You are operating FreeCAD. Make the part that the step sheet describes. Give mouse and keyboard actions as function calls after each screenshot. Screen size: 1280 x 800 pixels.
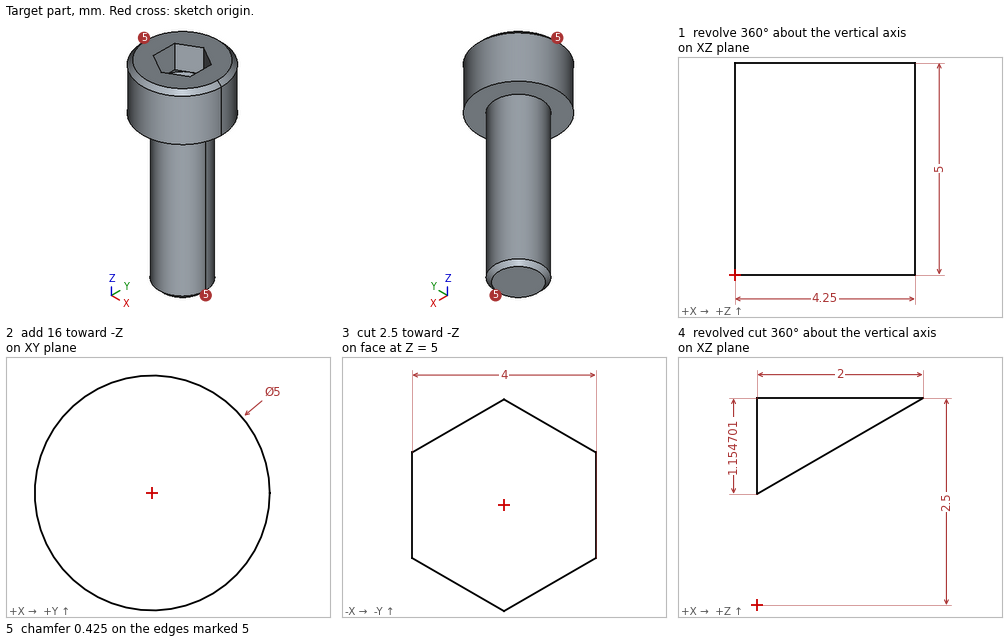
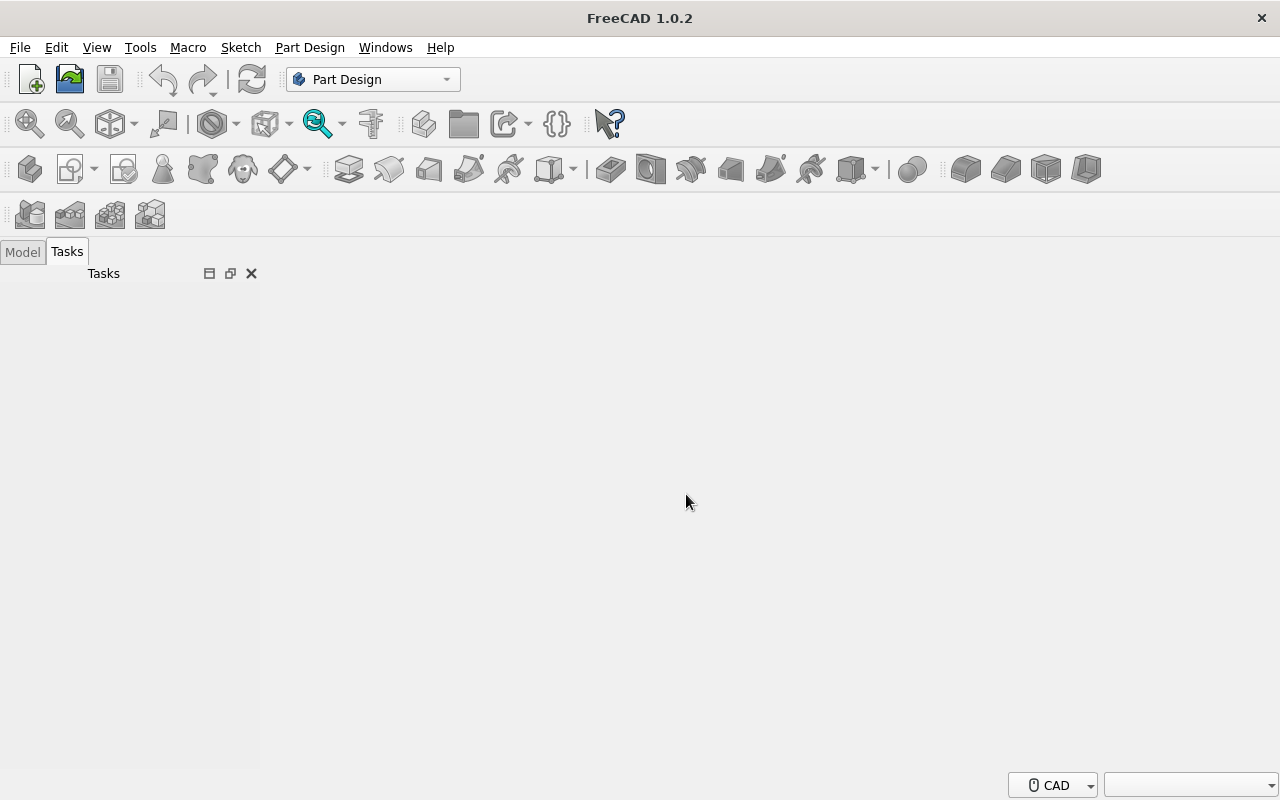
click(30, 80)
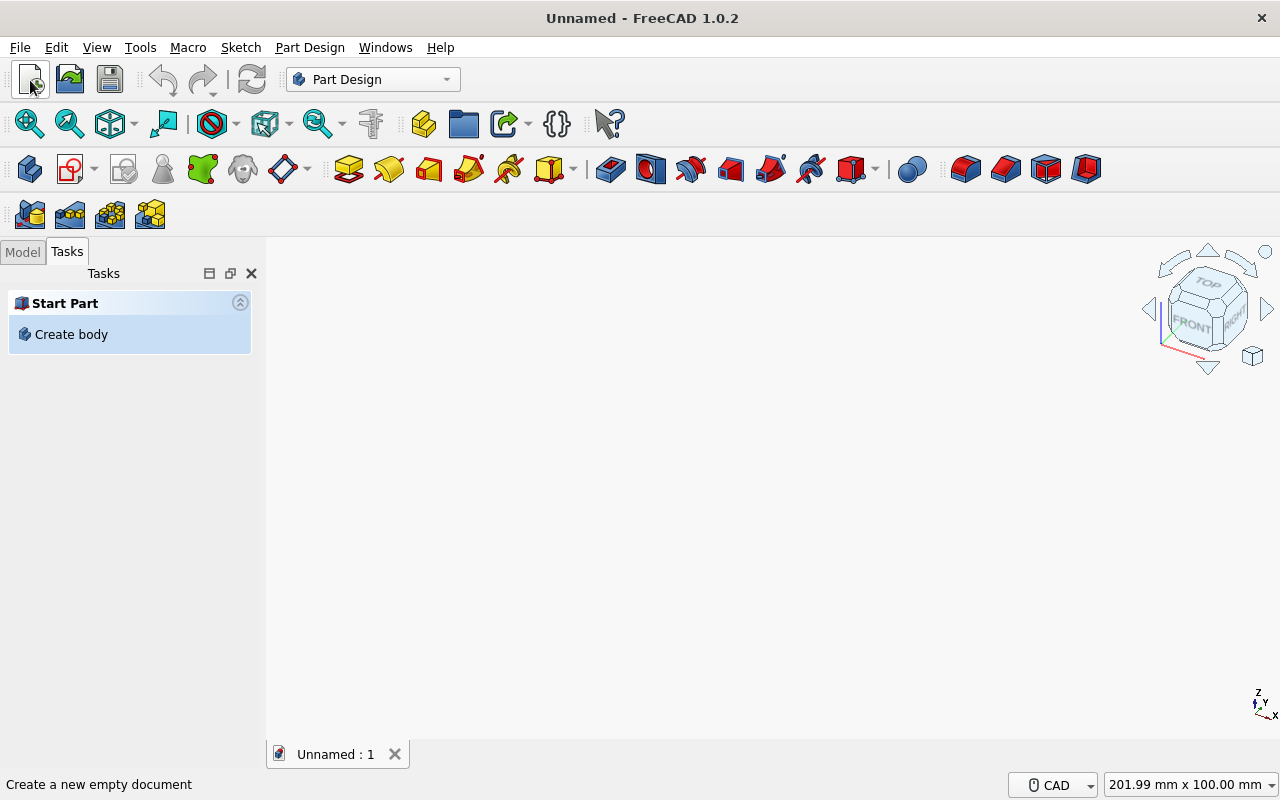
click(70, 170)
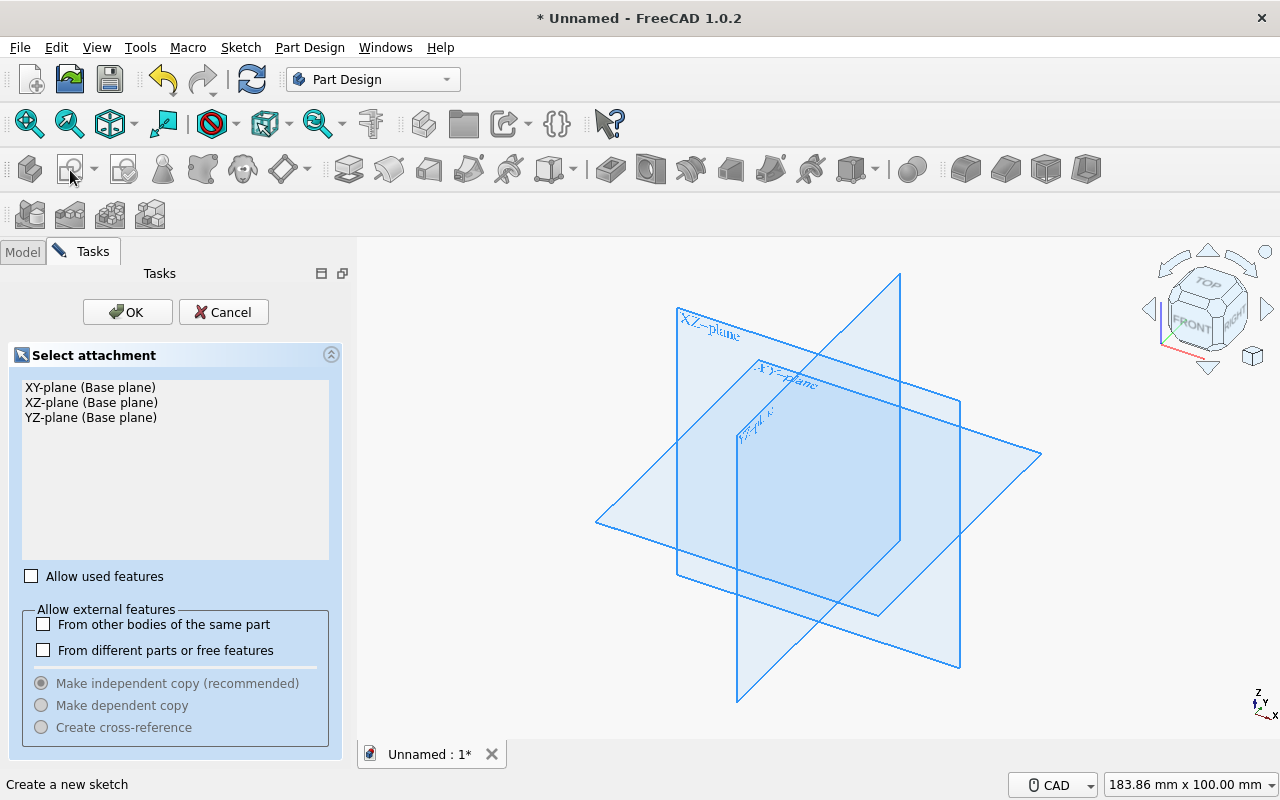
click(82, 402)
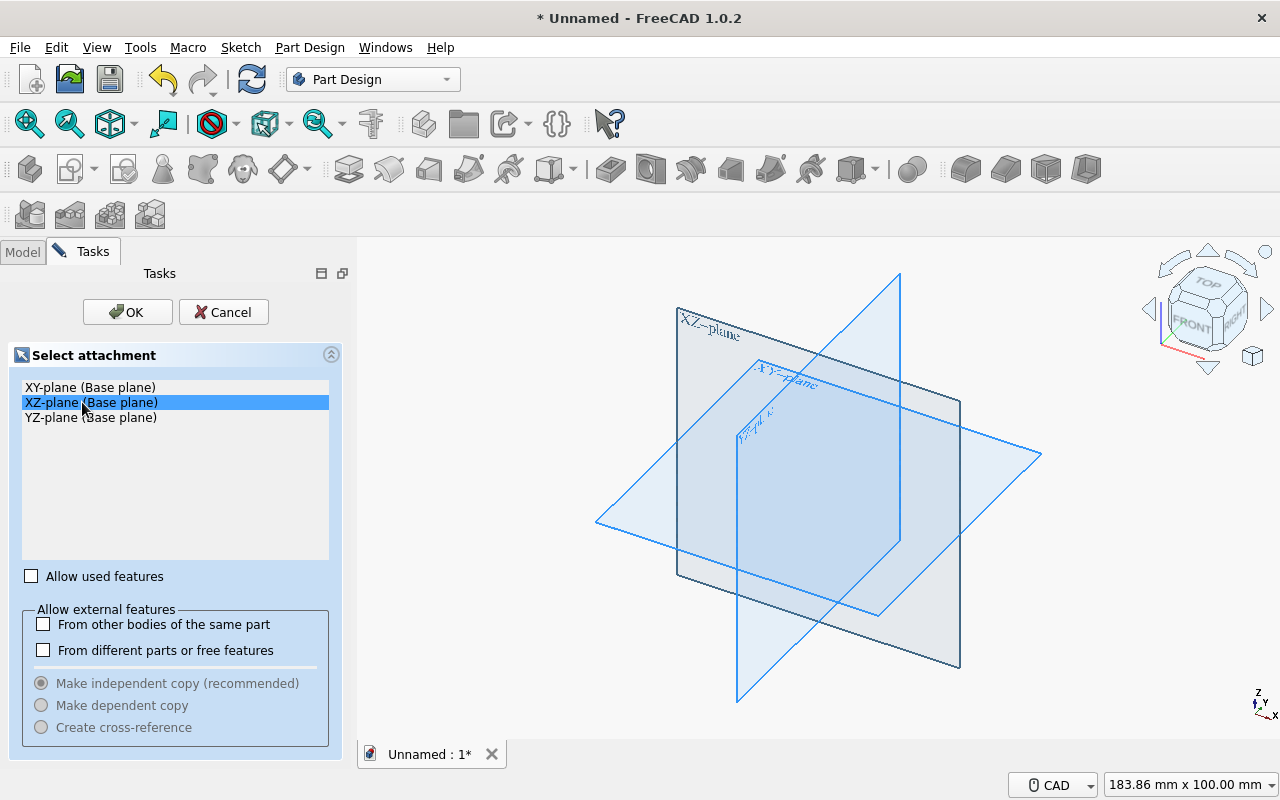
click(128, 312)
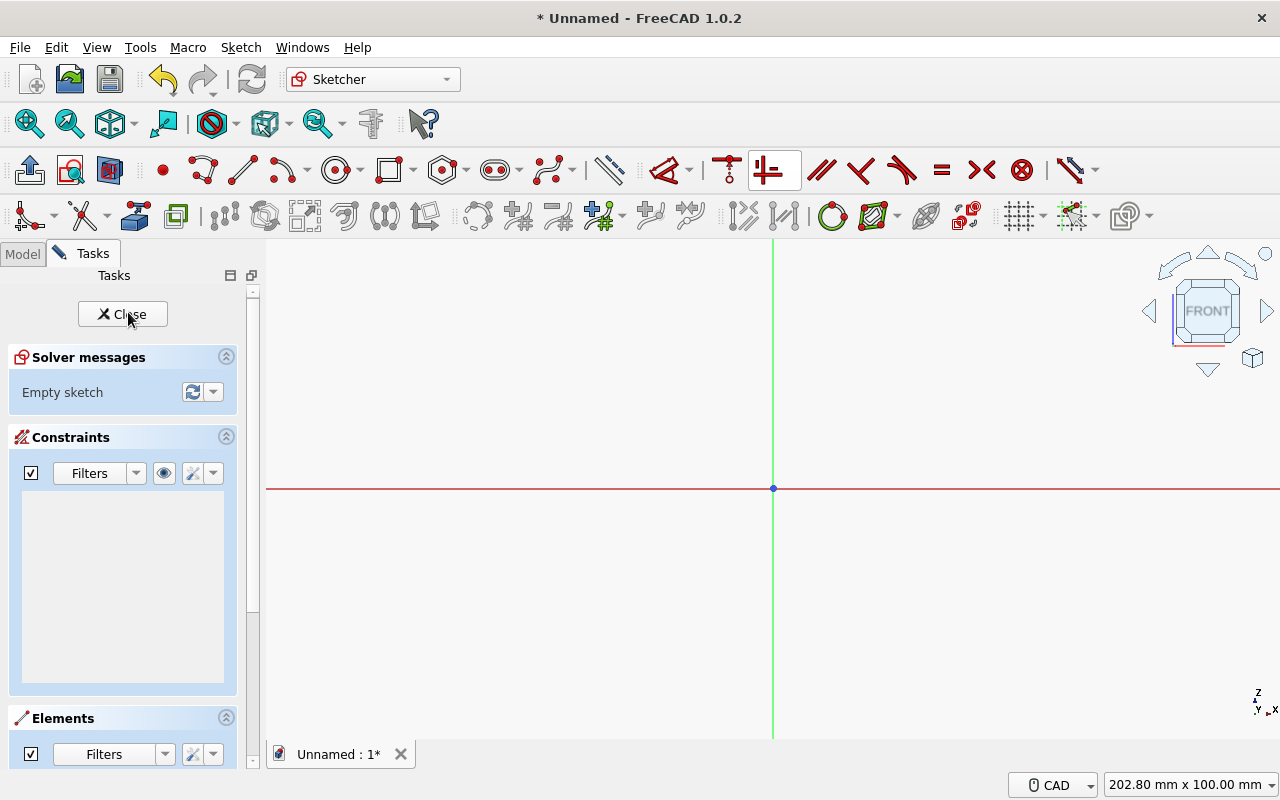
scroll(790, 475, up, 13)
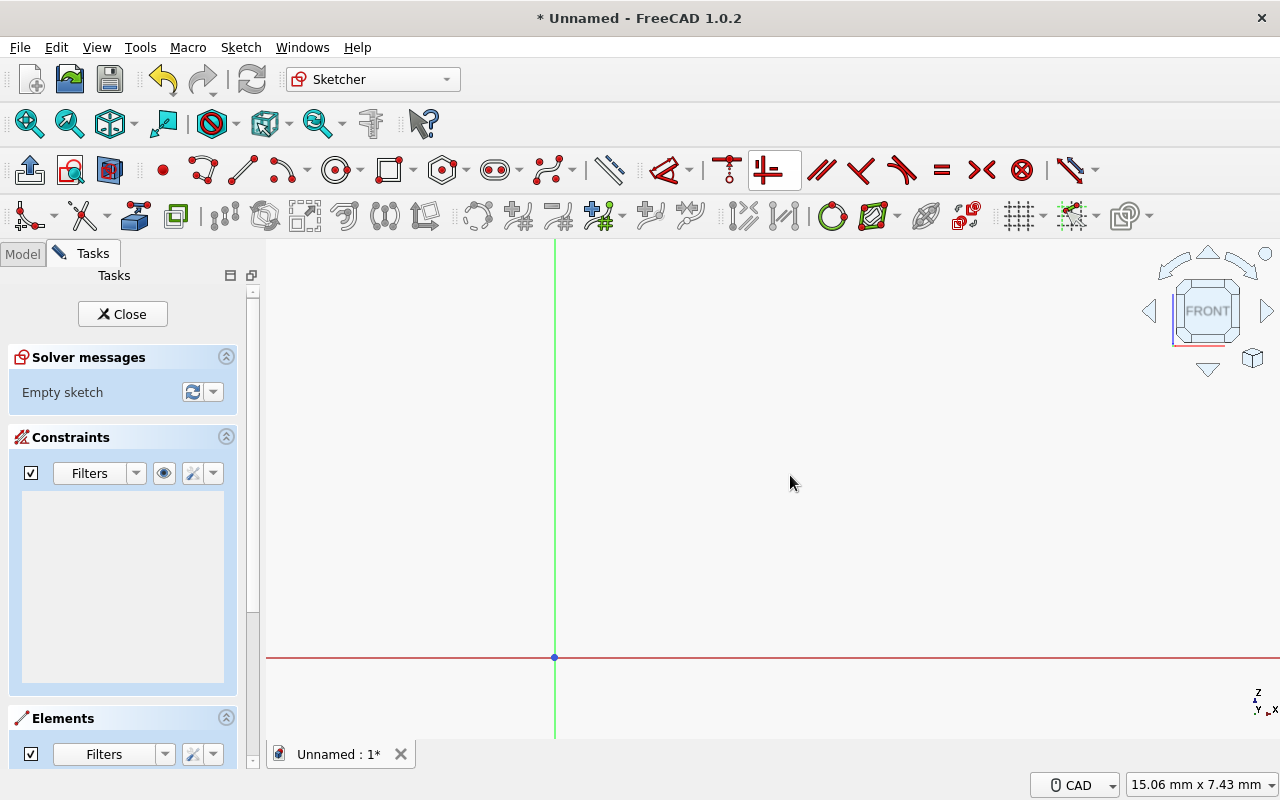
click(390, 170)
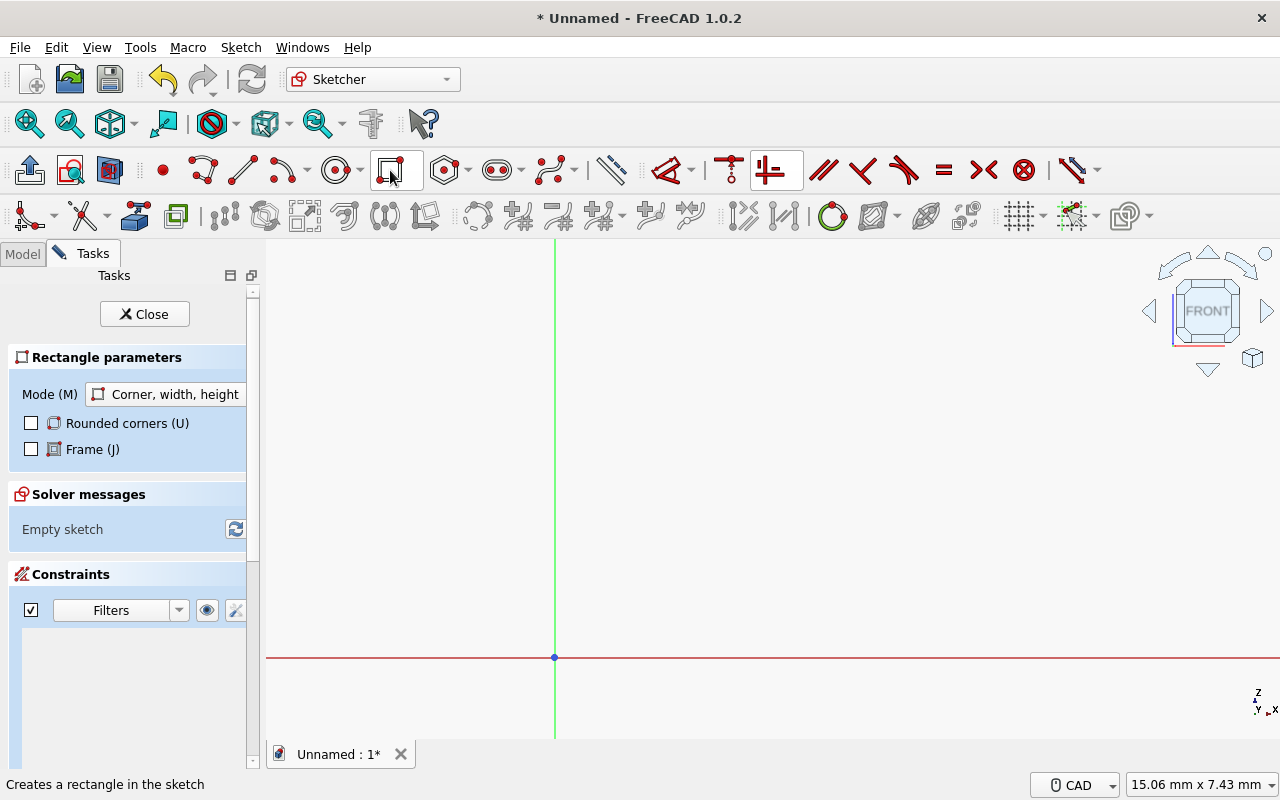
click(555, 658)
move(841, 321)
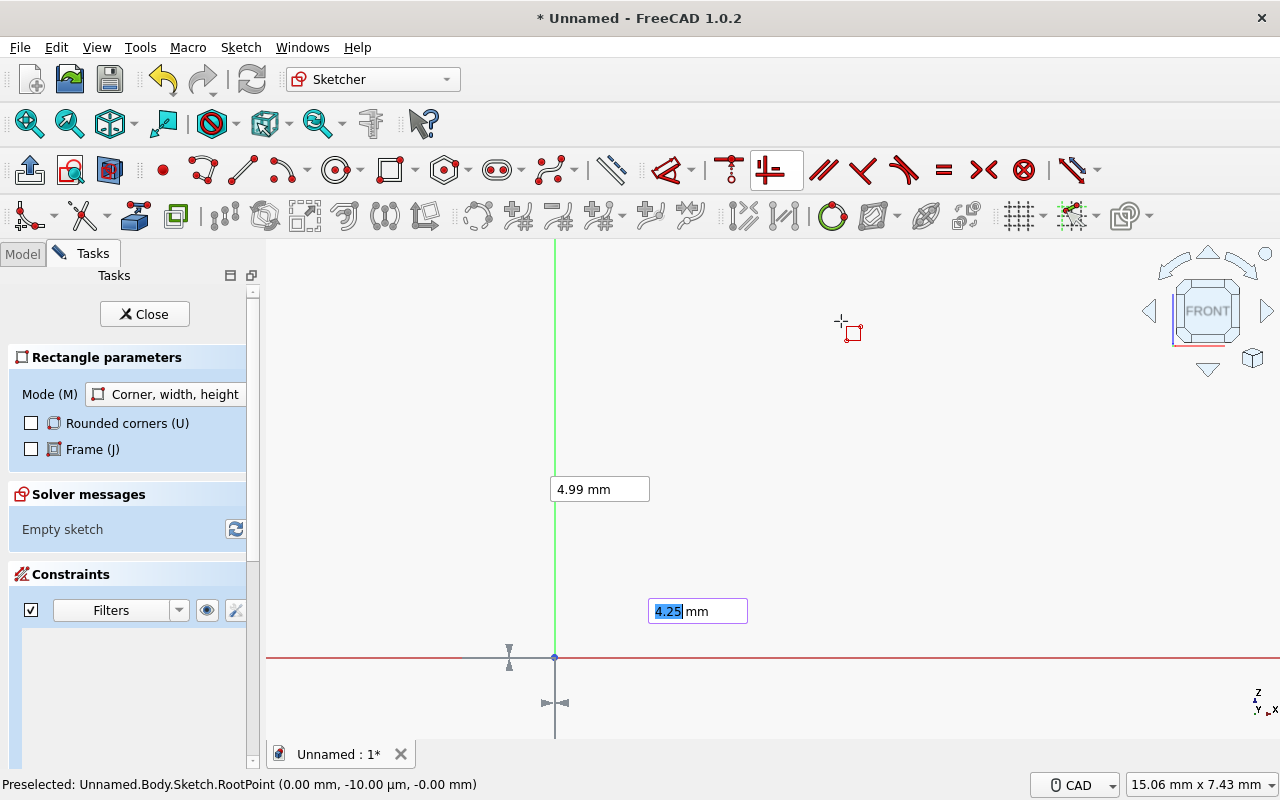
text(4.25)
key(Tab)
text(5)
key(Return)
key(Escape)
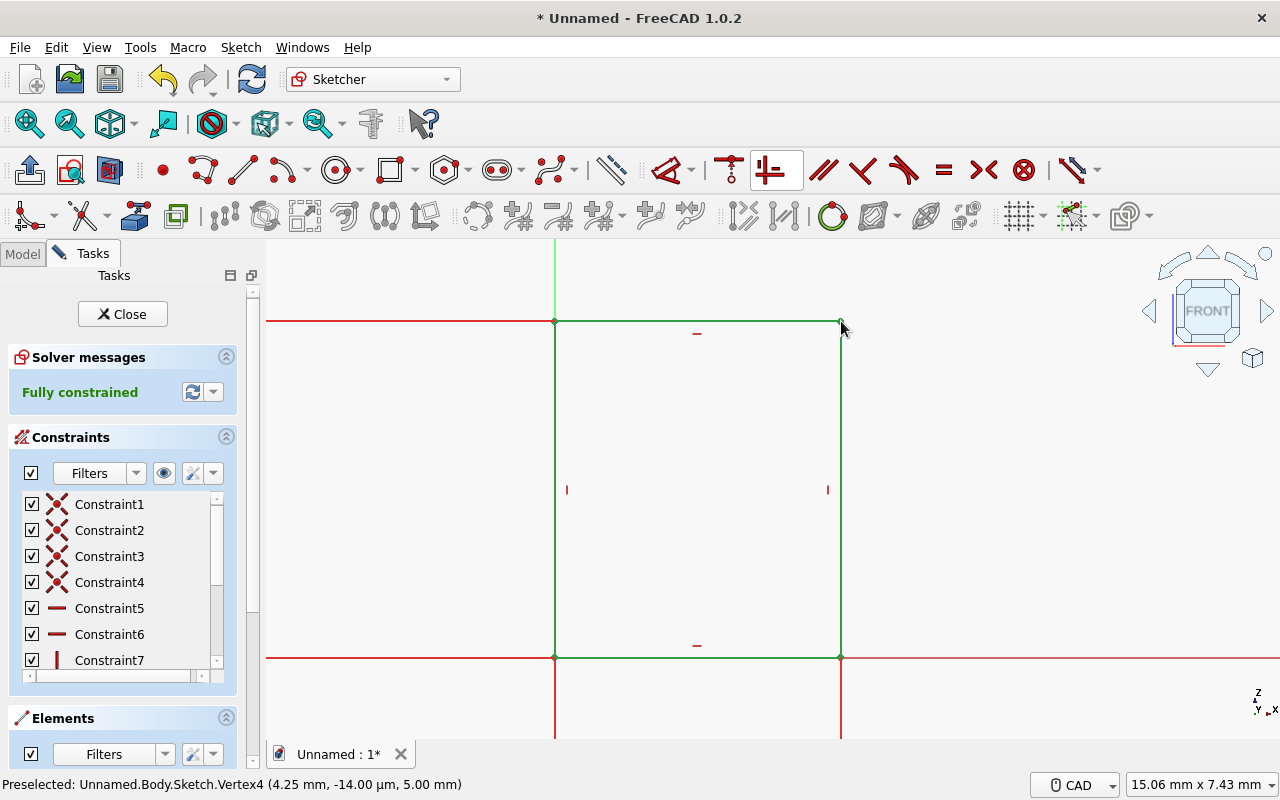
click(123, 314)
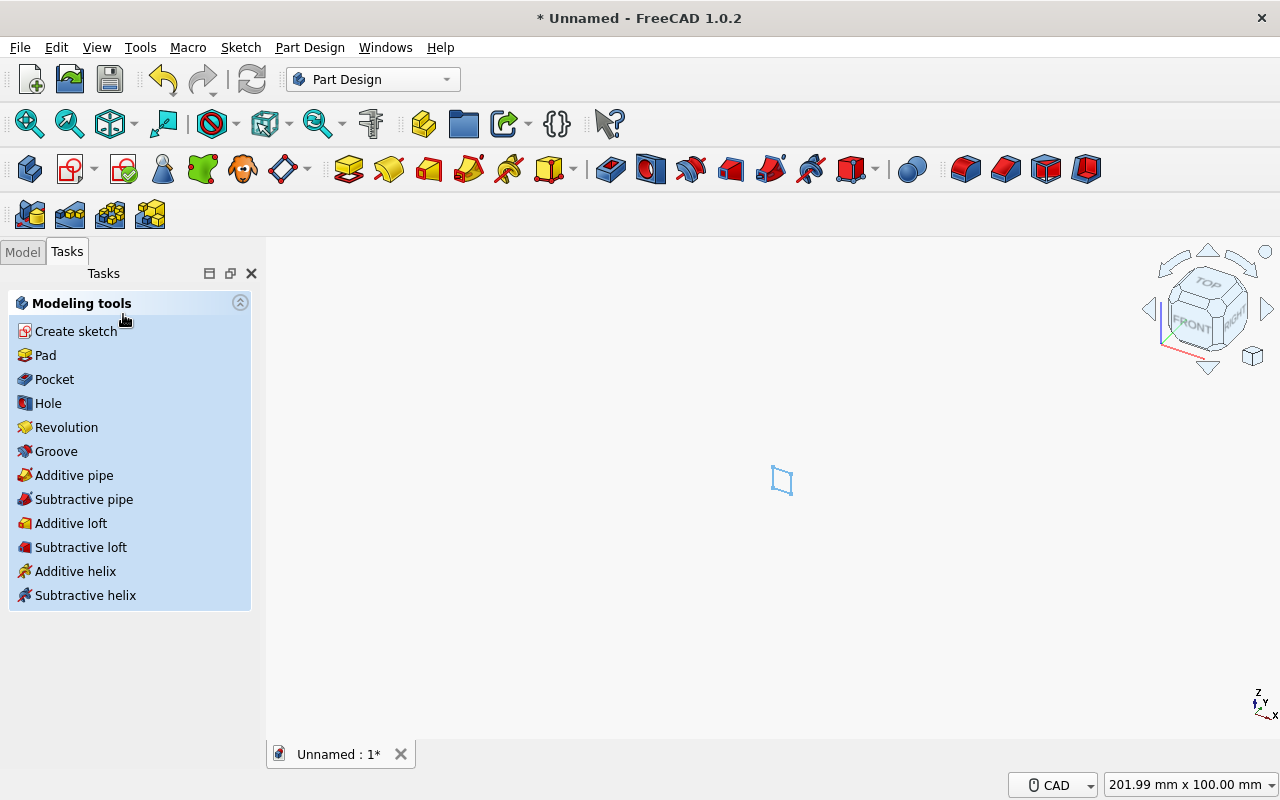
click(390, 170)